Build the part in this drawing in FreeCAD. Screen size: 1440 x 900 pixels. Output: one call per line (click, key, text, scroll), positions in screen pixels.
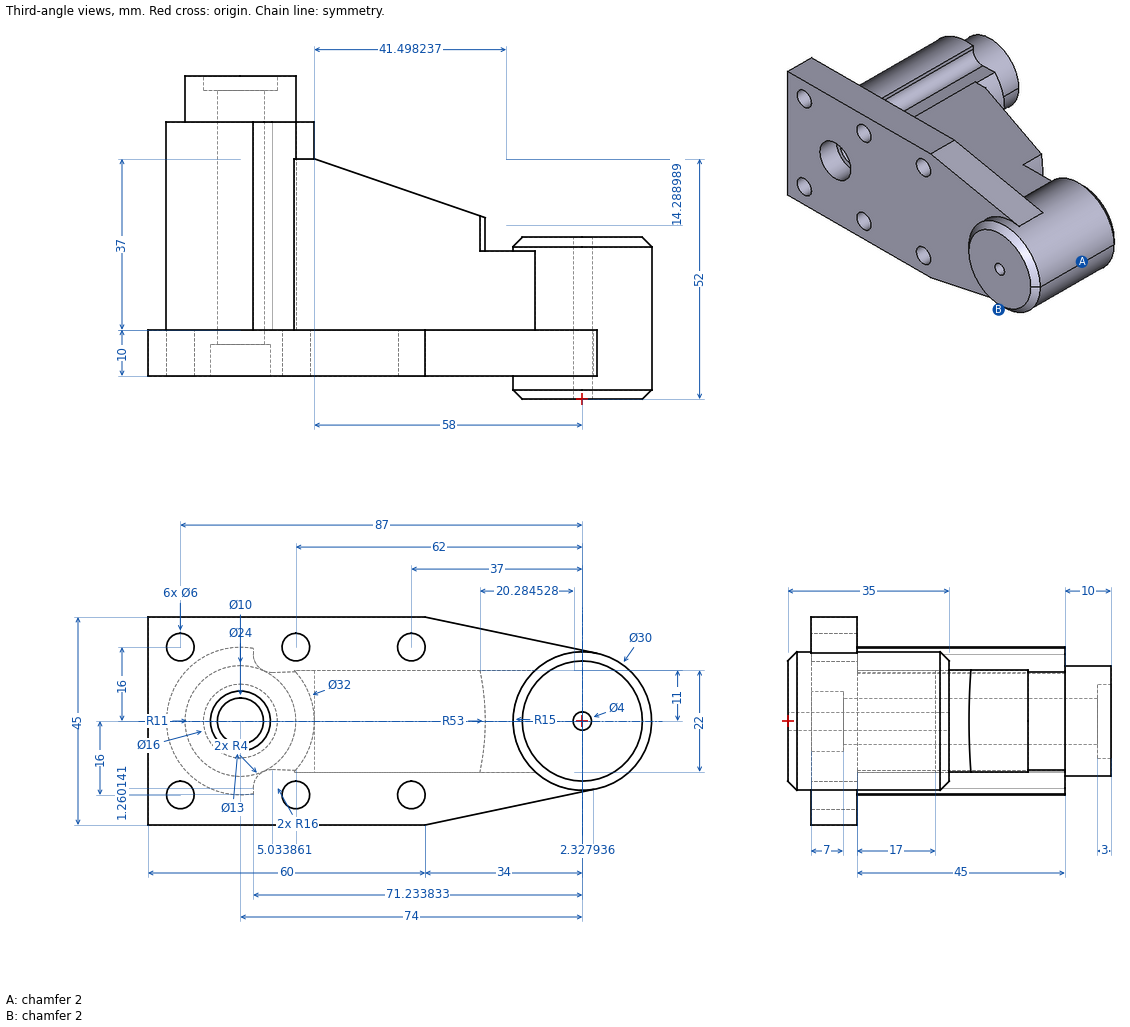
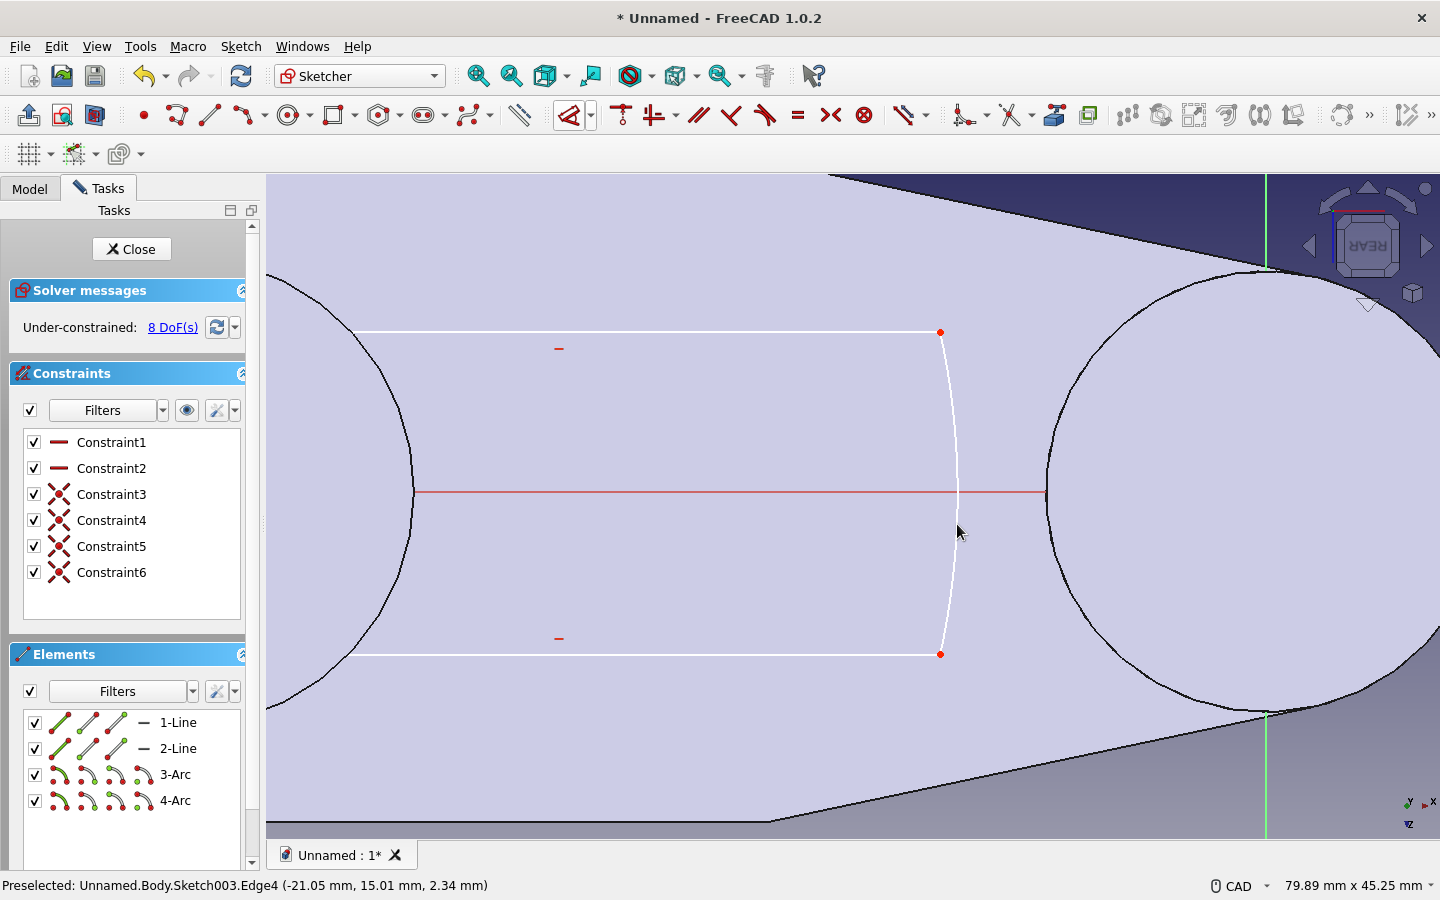
click(712, 332)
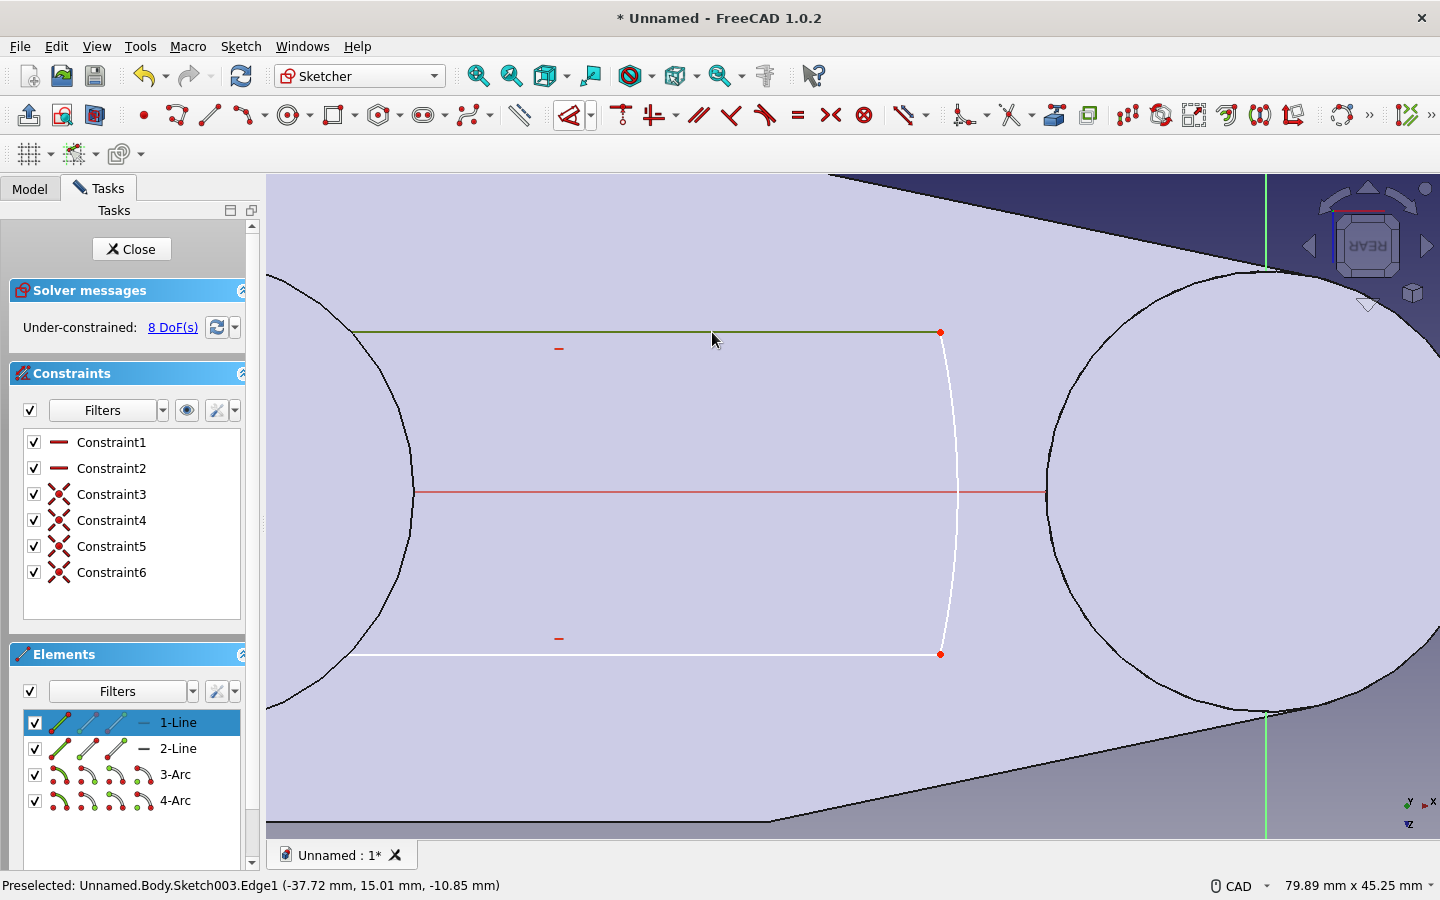
scroll(958, 525, down, 3)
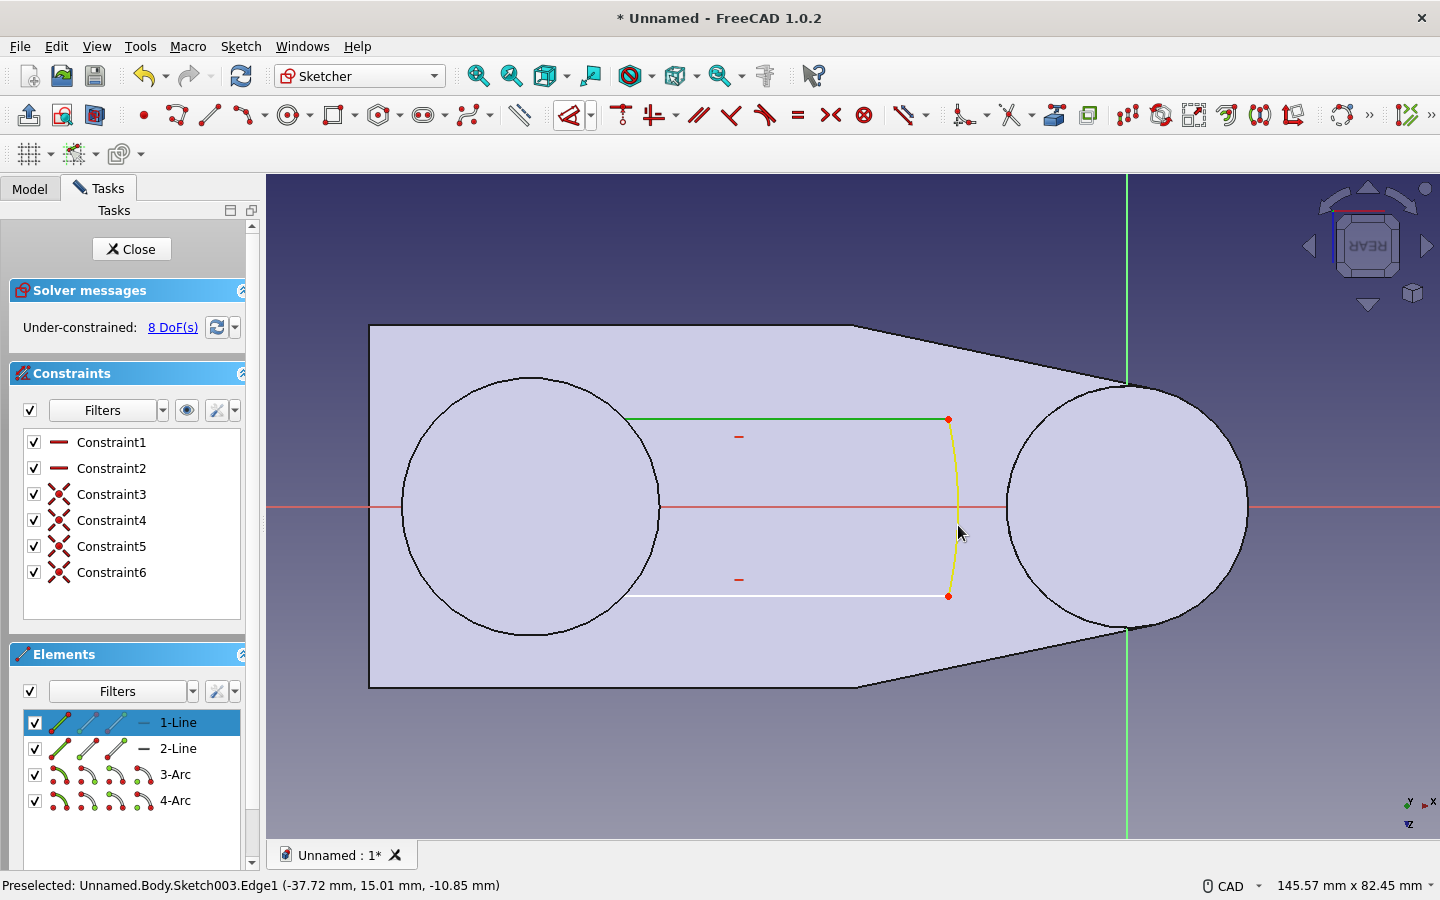
click(459, 456)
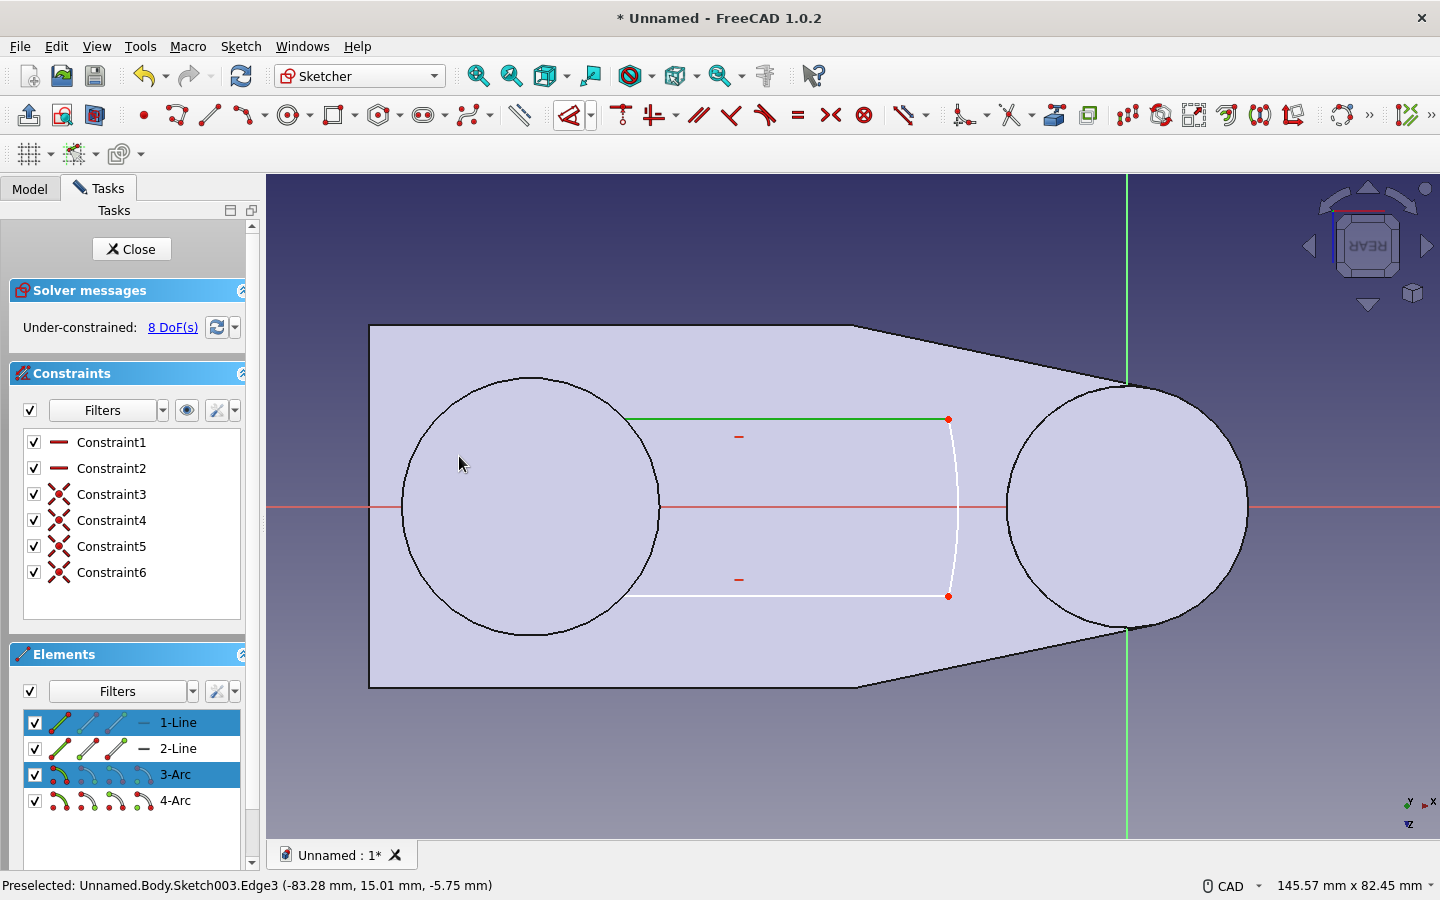
click(765, 116)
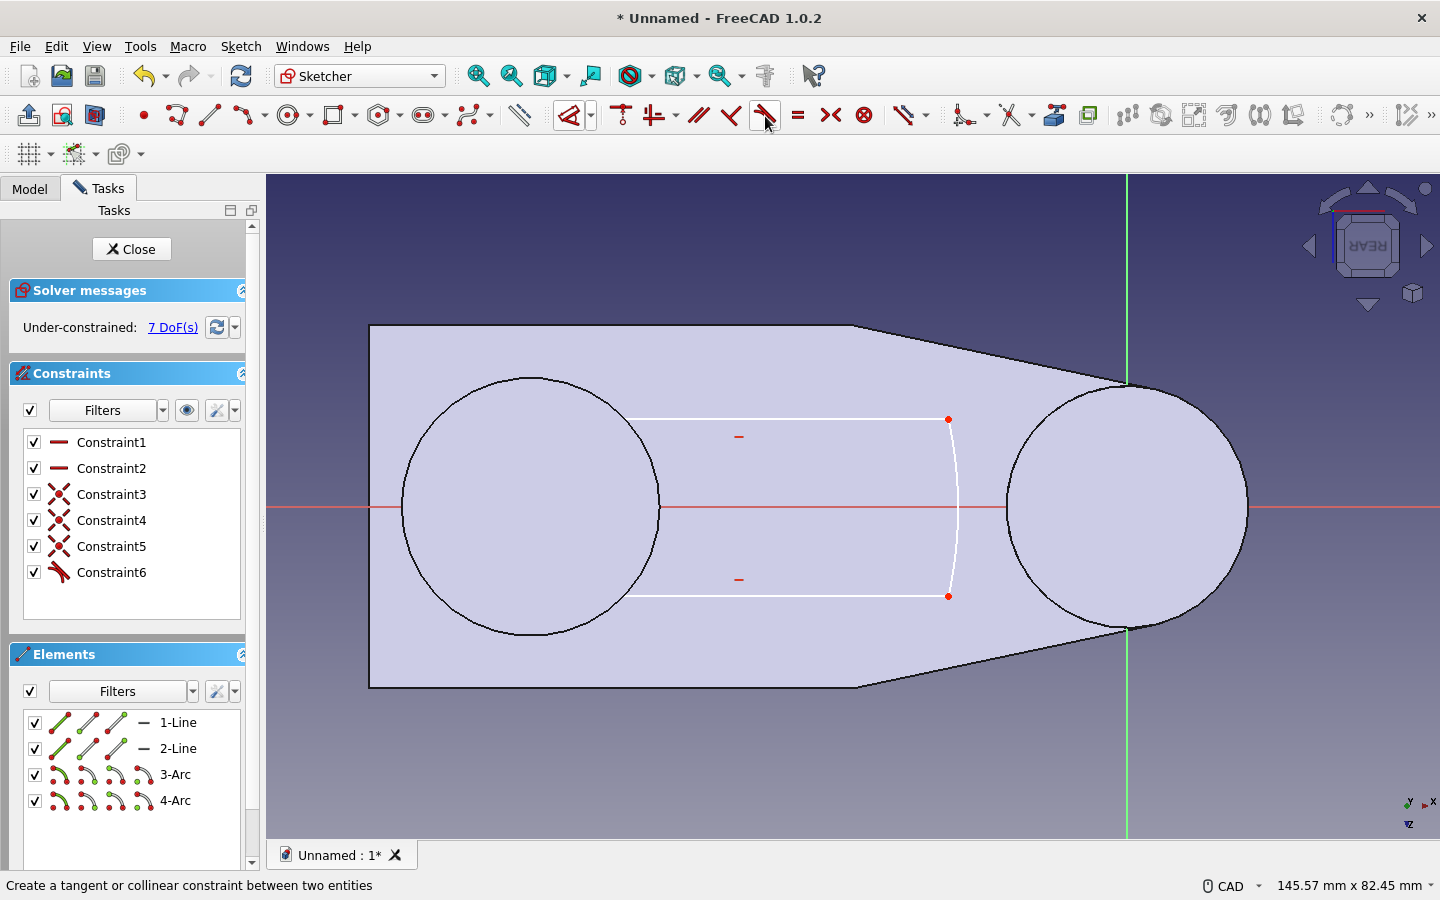
click(656, 596)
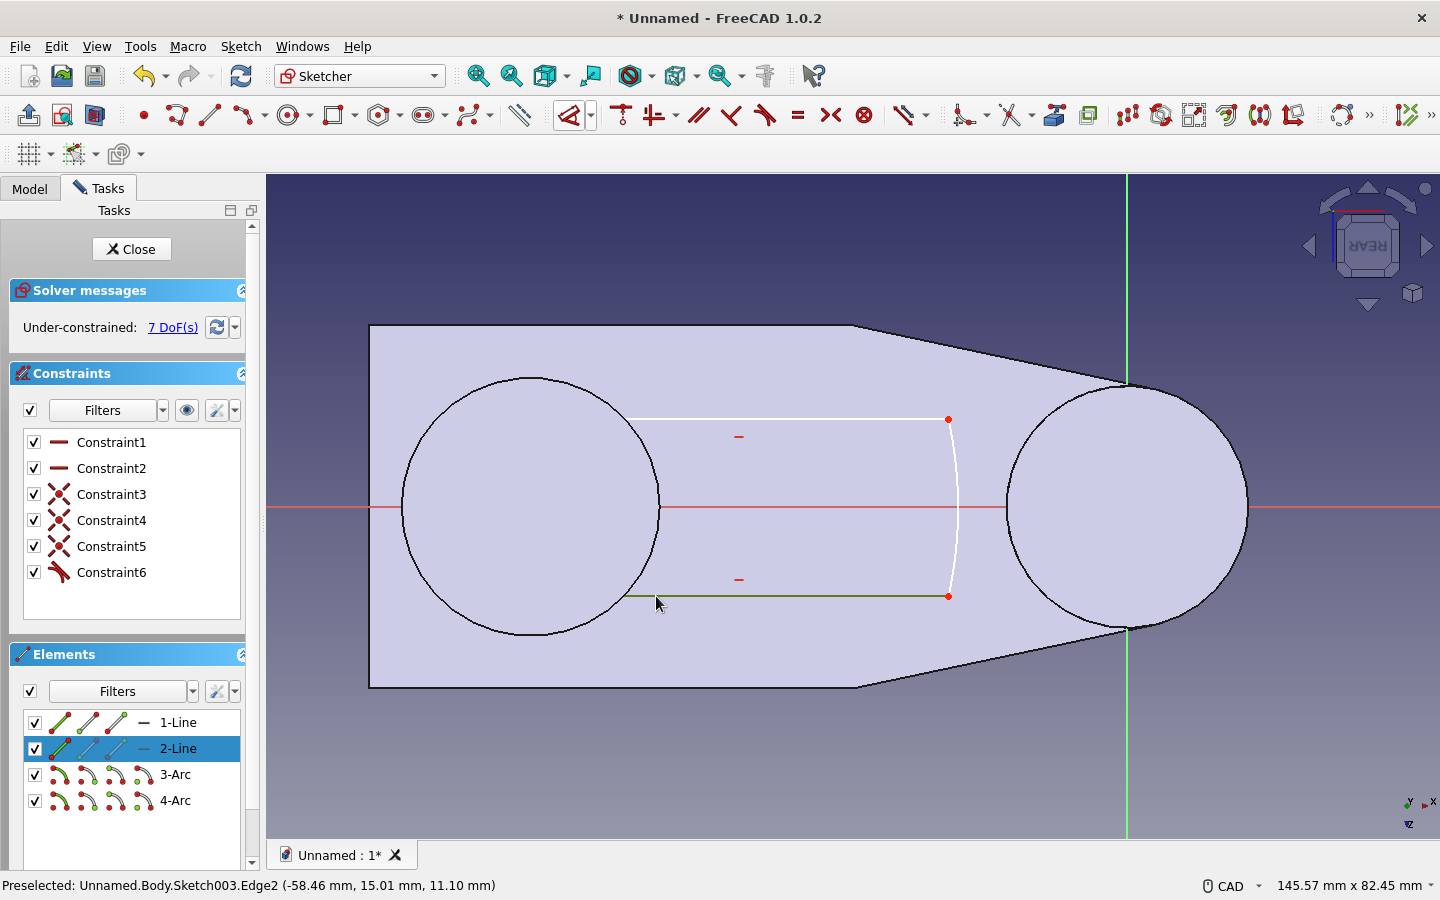
click(459, 456)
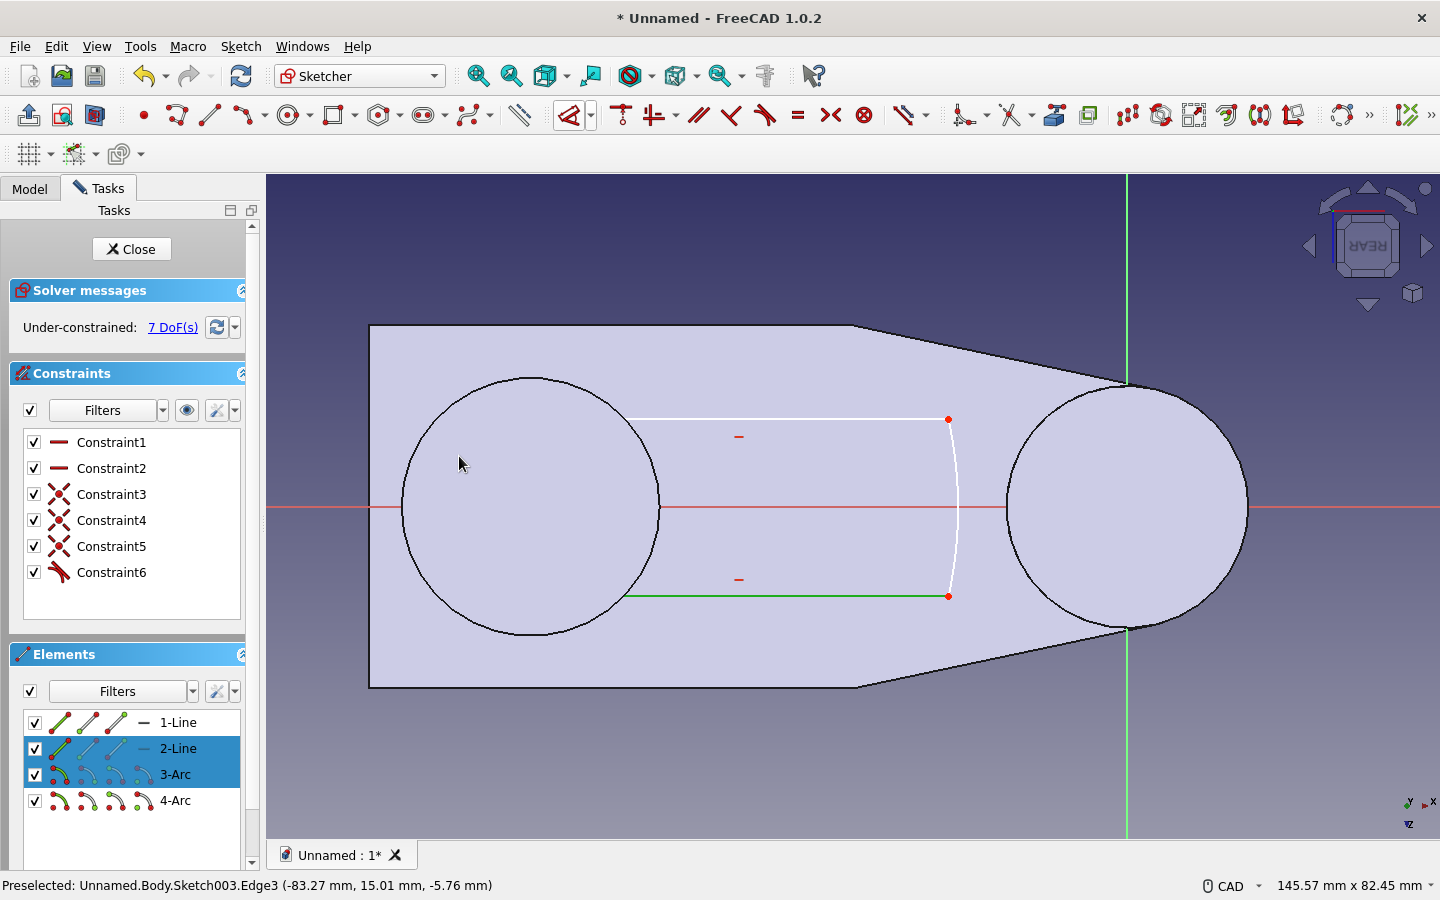
click(765, 116)